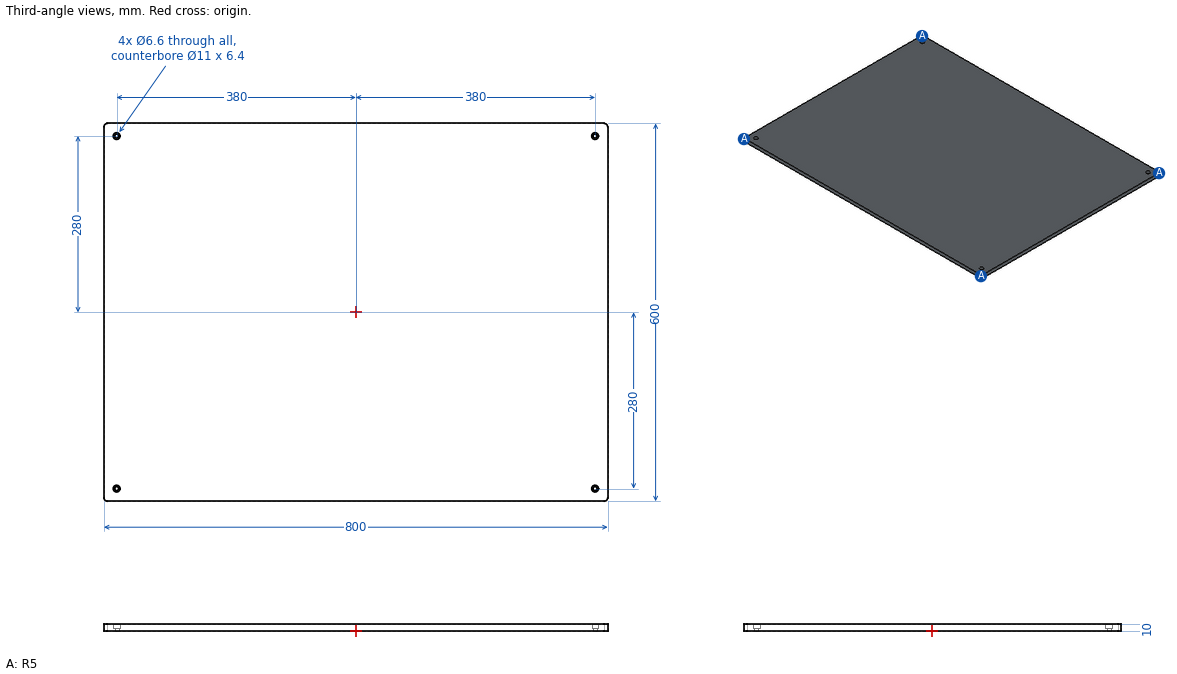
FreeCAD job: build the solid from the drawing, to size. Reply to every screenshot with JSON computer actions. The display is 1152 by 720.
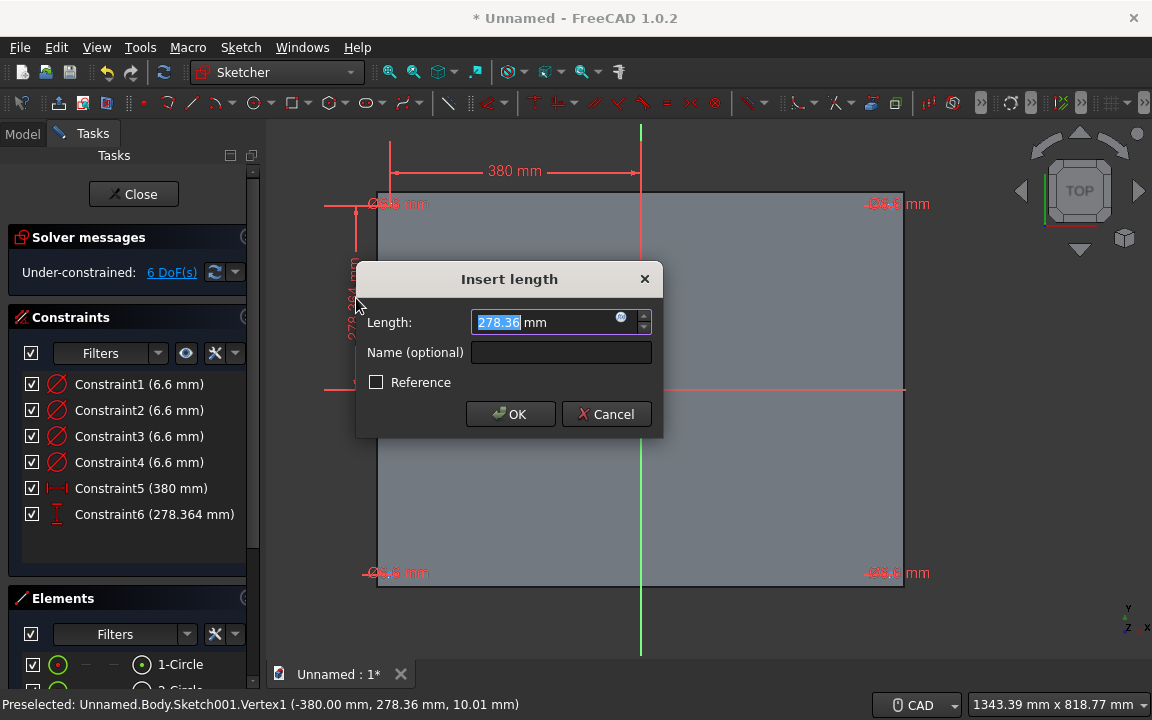
{"action": "type", "text": "280"}
{"action": "key", "text": "Return"}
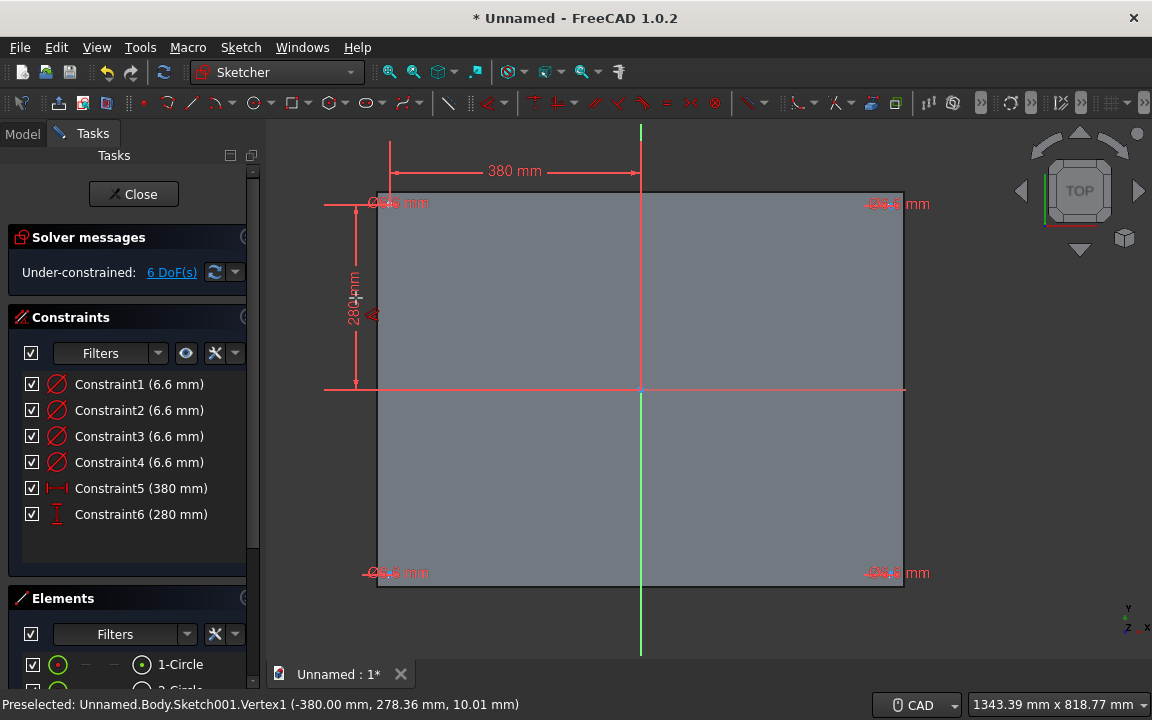
{"action": "left_click", "coordinate": [891, 206]}
{"action": "left_click", "coordinate": [766, 172]}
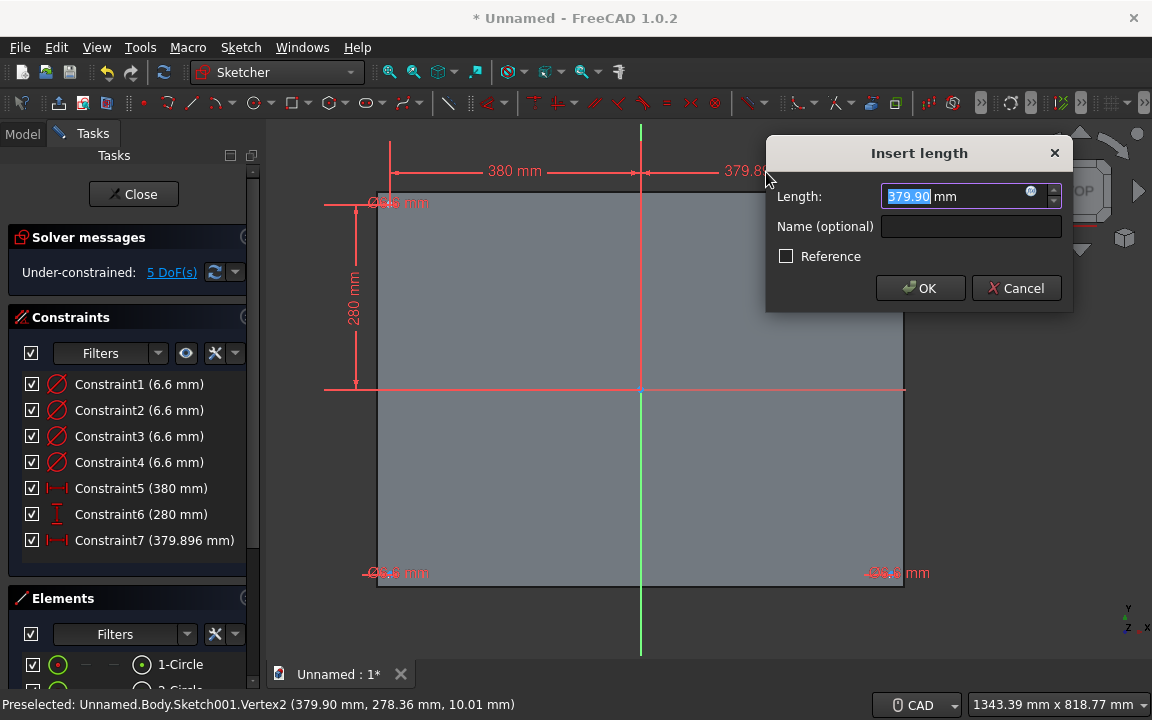
{"action": "type", "text": "380"}
{"action": "key", "text": "Return"}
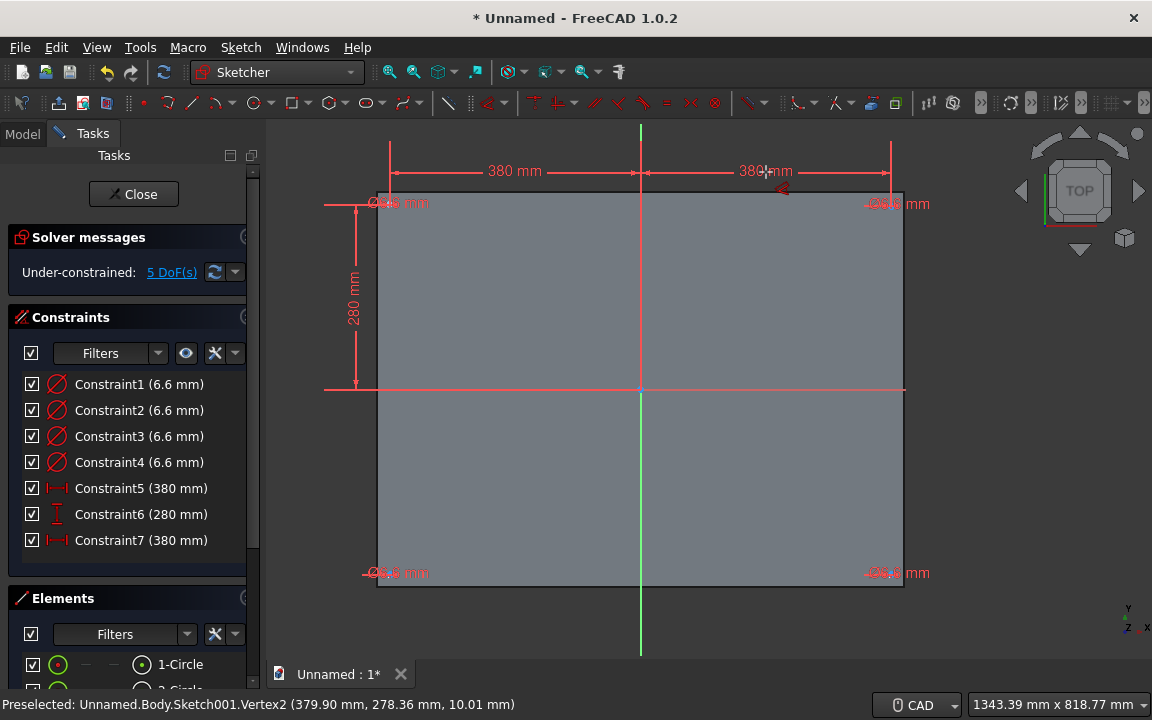
{"action": "left_click", "coordinate": [891, 206]}
{"action": "left_click", "coordinate": [925, 298]}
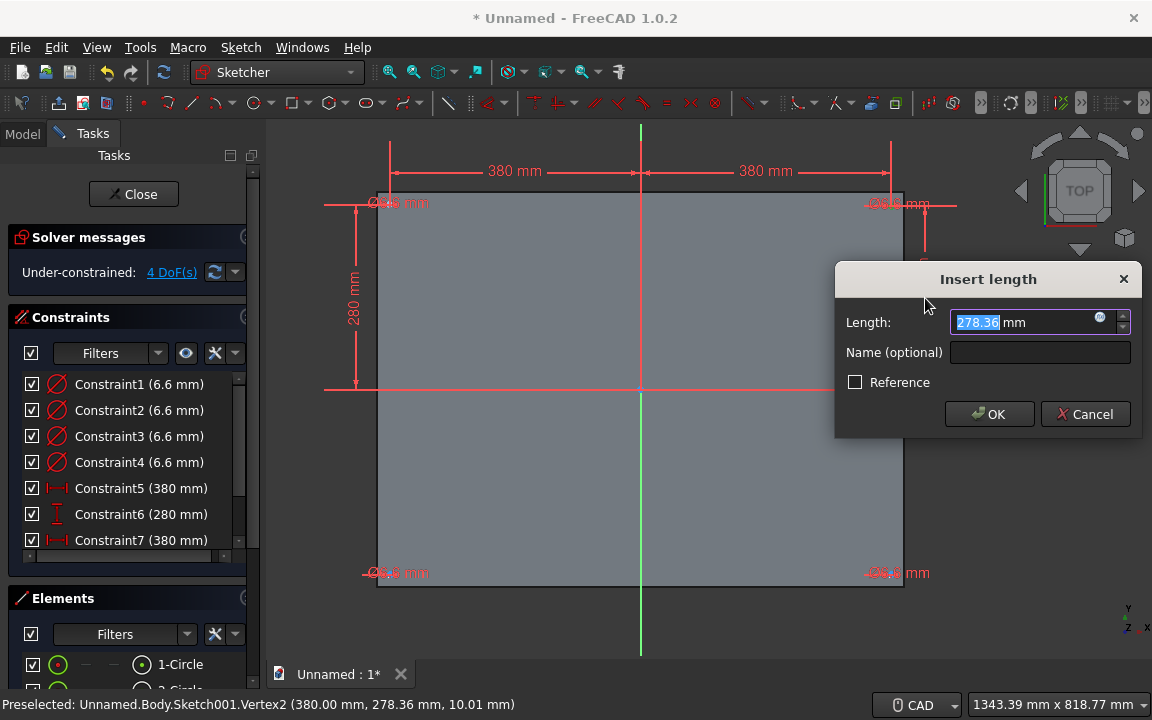
{"action": "type", "text": "280"}
{"action": "key", "text": "Return"}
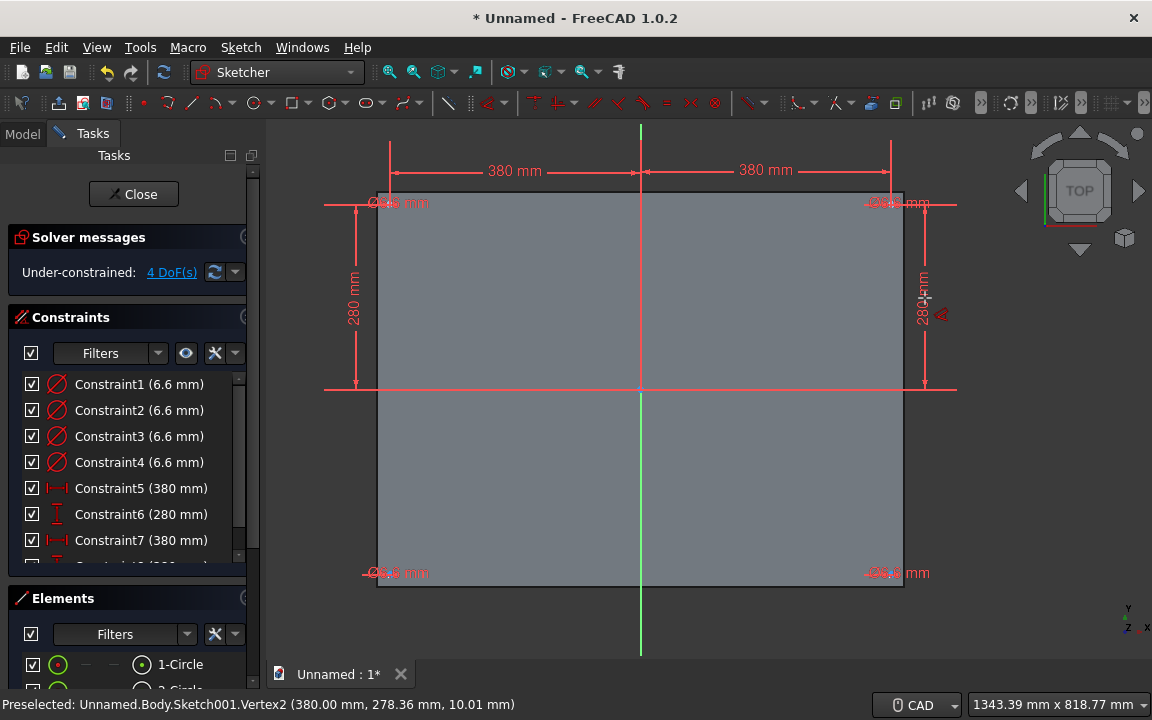
{"action": "left_click", "coordinate": [891, 575]}
{"action": "left_click", "coordinate": [766, 609]}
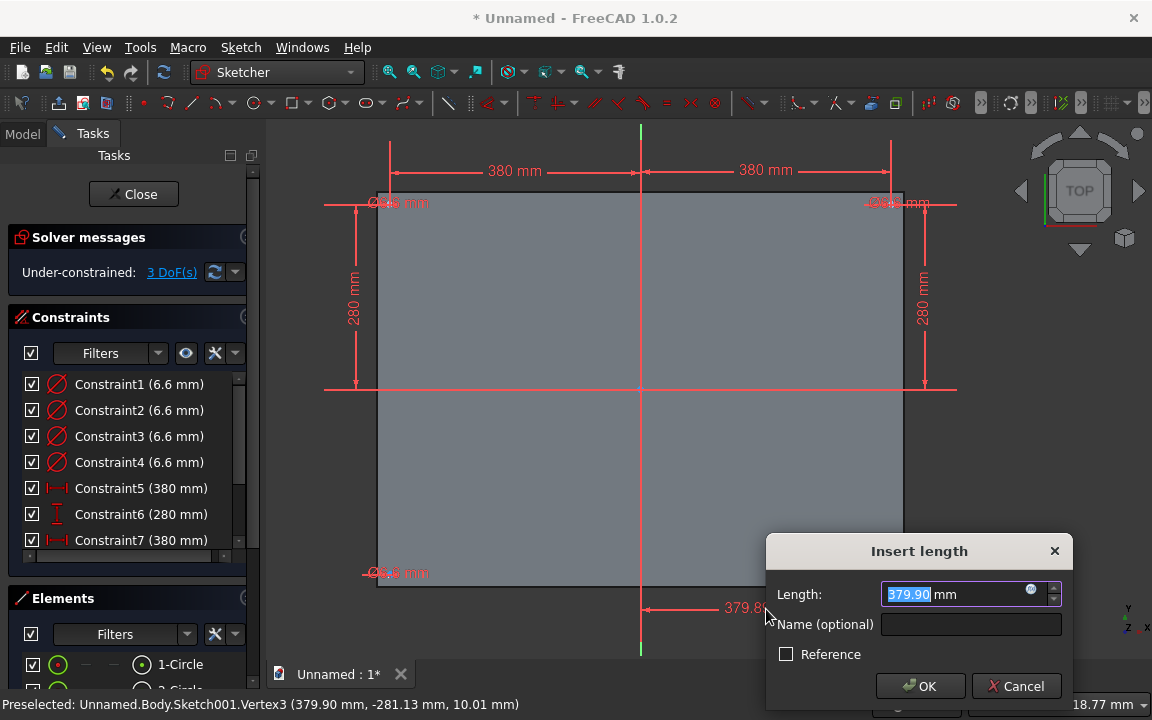
{"action": "type", "text": "380"}
{"action": "key", "text": "Return"}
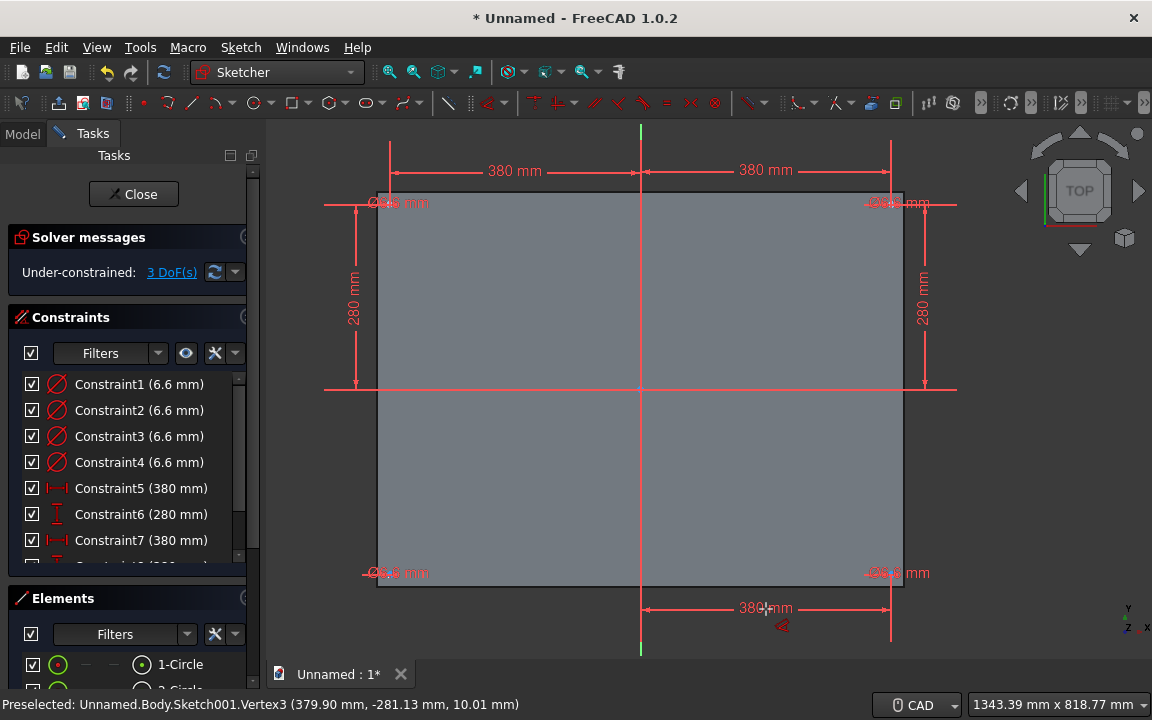
{"action": "left_click", "coordinate": [891, 575]}
{"action": "left_click", "coordinate": [925, 482]}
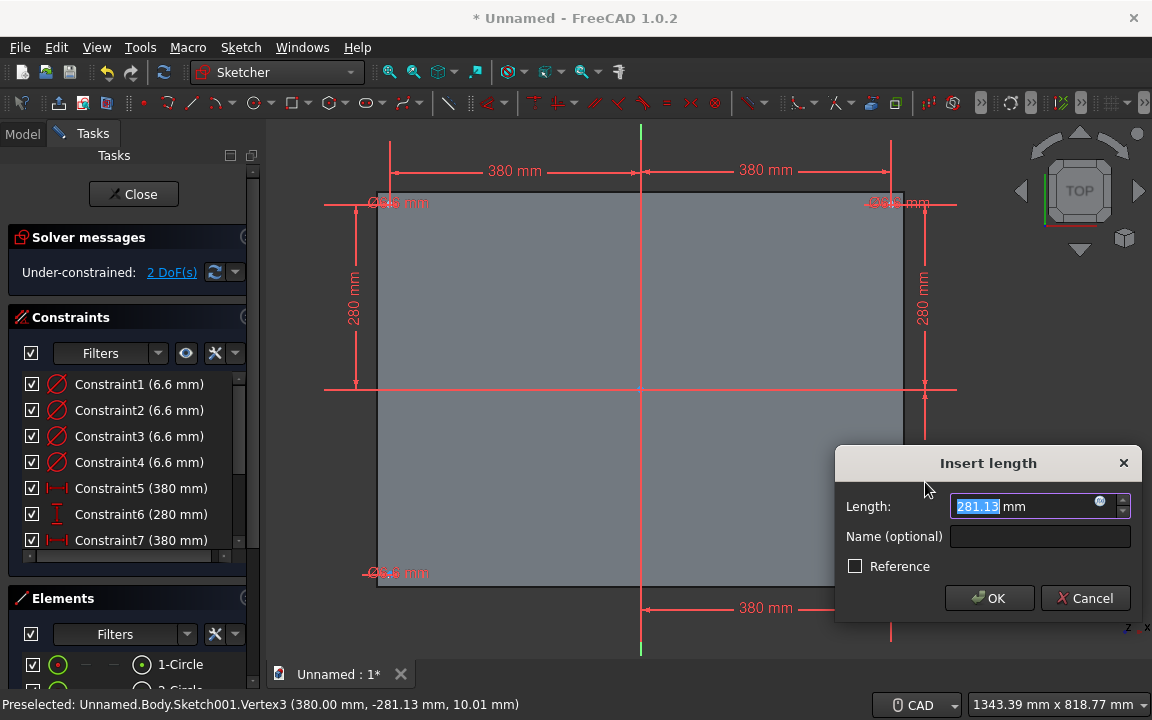
{"action": "type", "text": "280"}
{"action": "key", "text": "Return"}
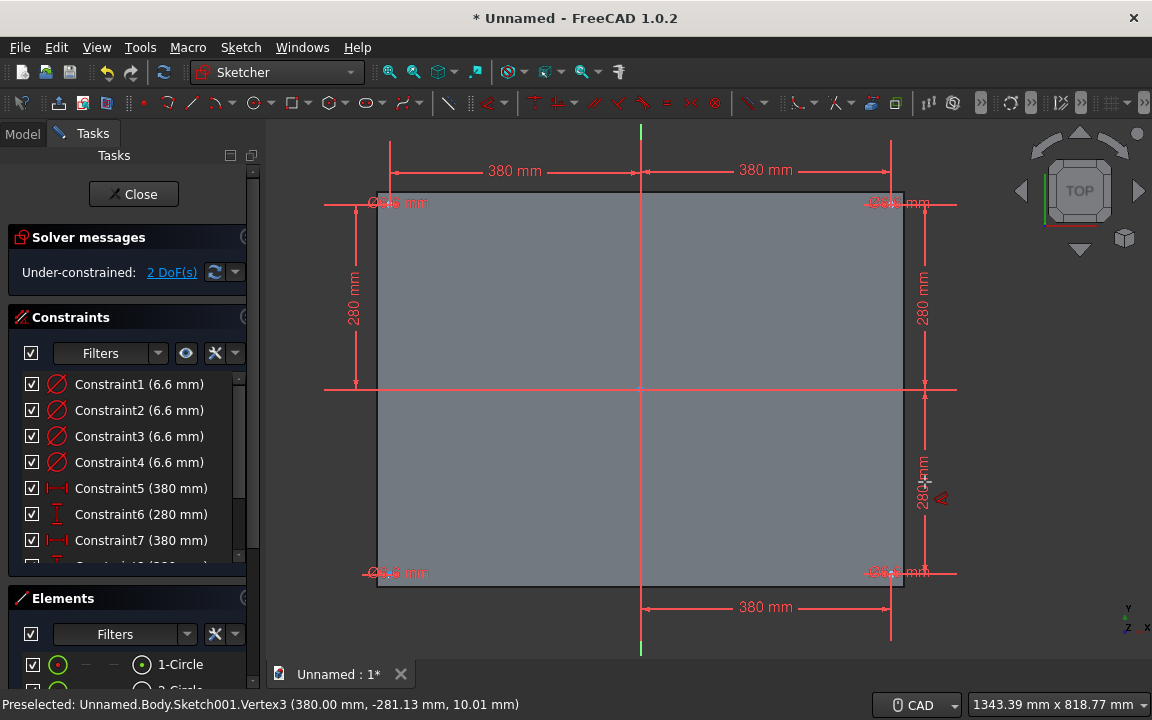
{"action": "left_click", "coordinate": [390, 575]}
{"action": "left_click", "coordinate": [515, 609]}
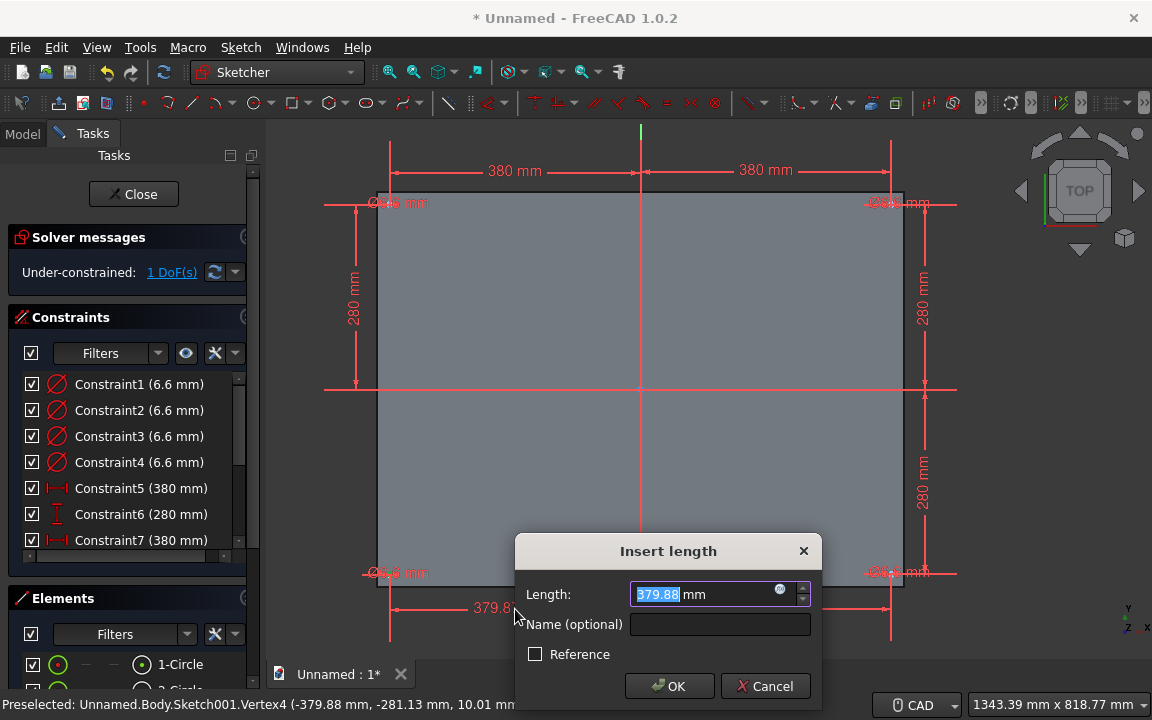
{"action": "type", "text": "380"}
{"action": "key", "text": "Return"}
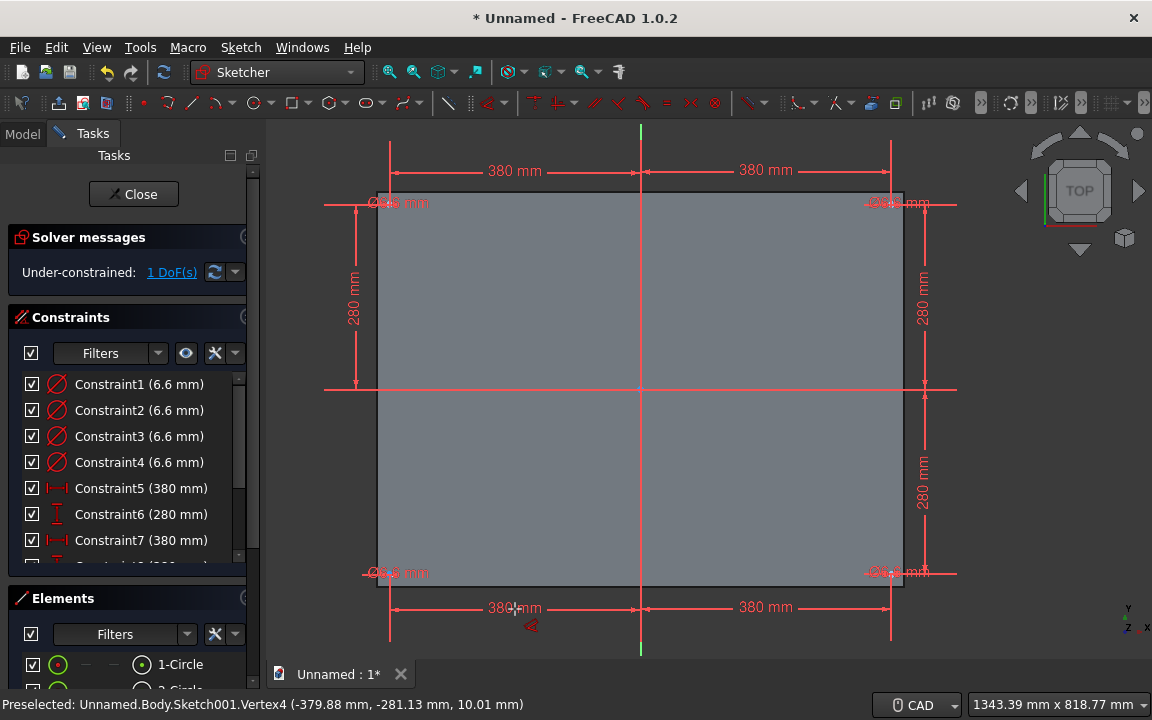
{"action": "left_click", "coordinate": [390, 575]}
{"action": "left_click", "coordinate": [356, 482]}